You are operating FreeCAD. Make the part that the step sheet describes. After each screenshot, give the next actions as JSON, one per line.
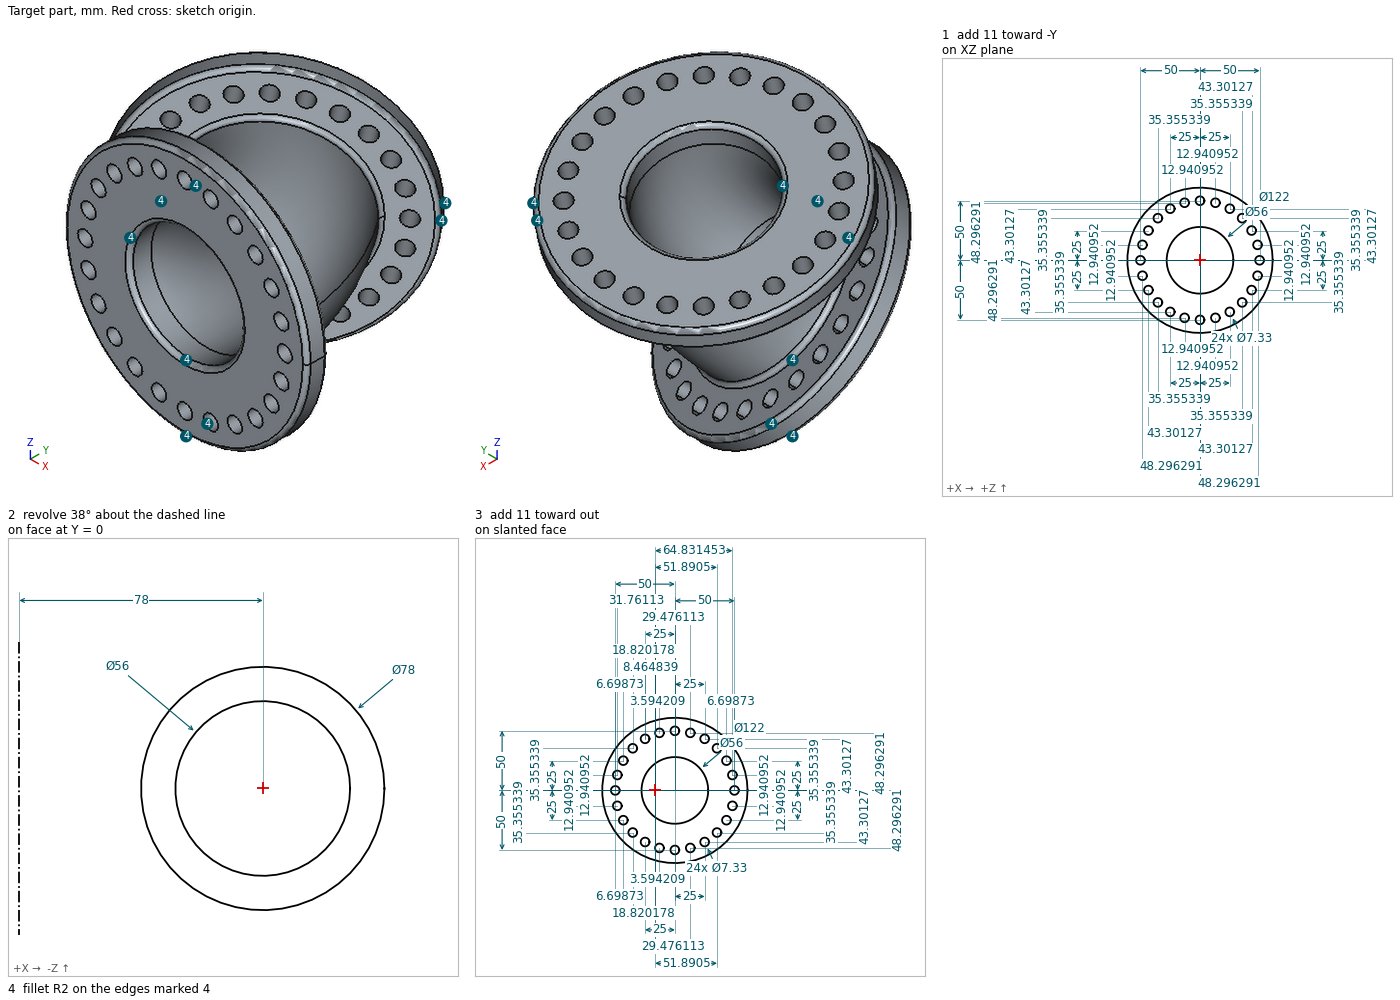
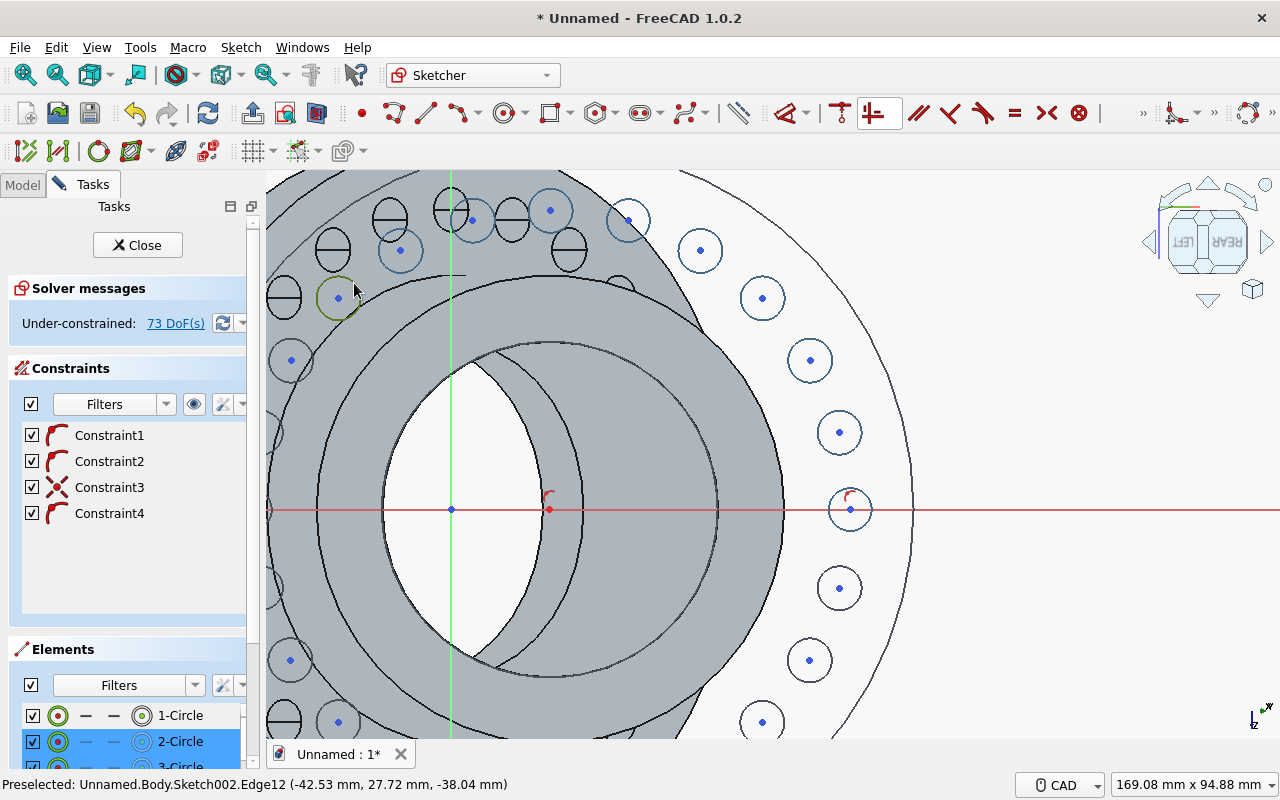
{"action": "left_click", "coordinate": [307, 345]}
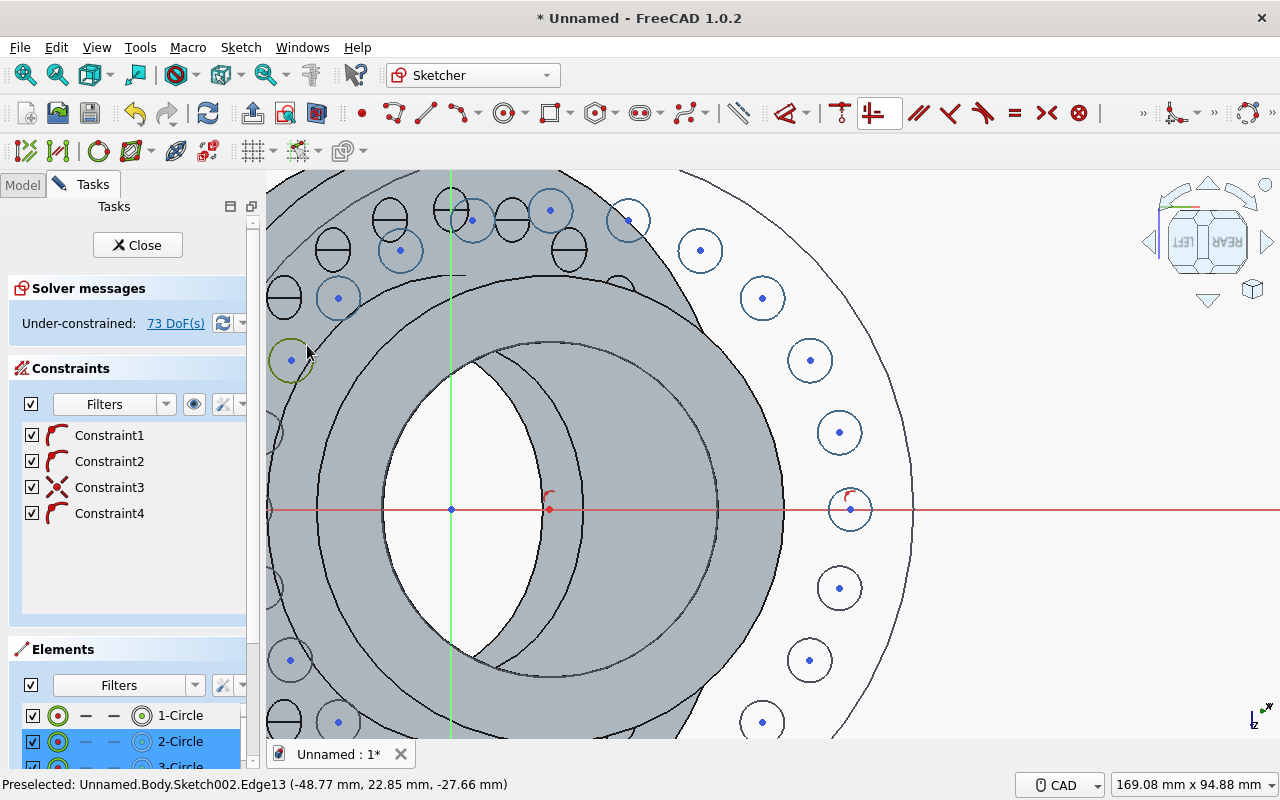
{"action": "scroll", "coordinate": [830, 410], "scroll_direction": "down", "scroll_amount": 4}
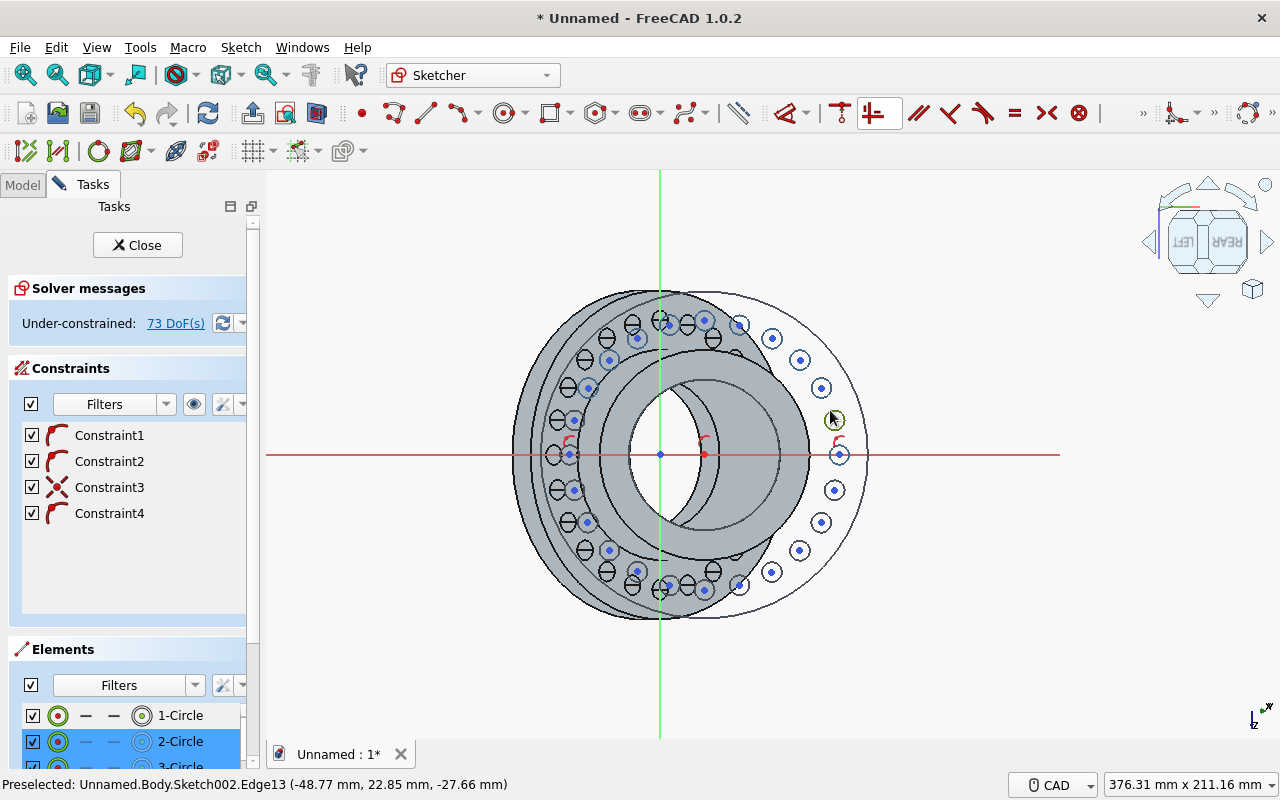
{"action": "scroll", "coordinate": [582, 413], "scroll_direction": "up", "scroll_amount": 2}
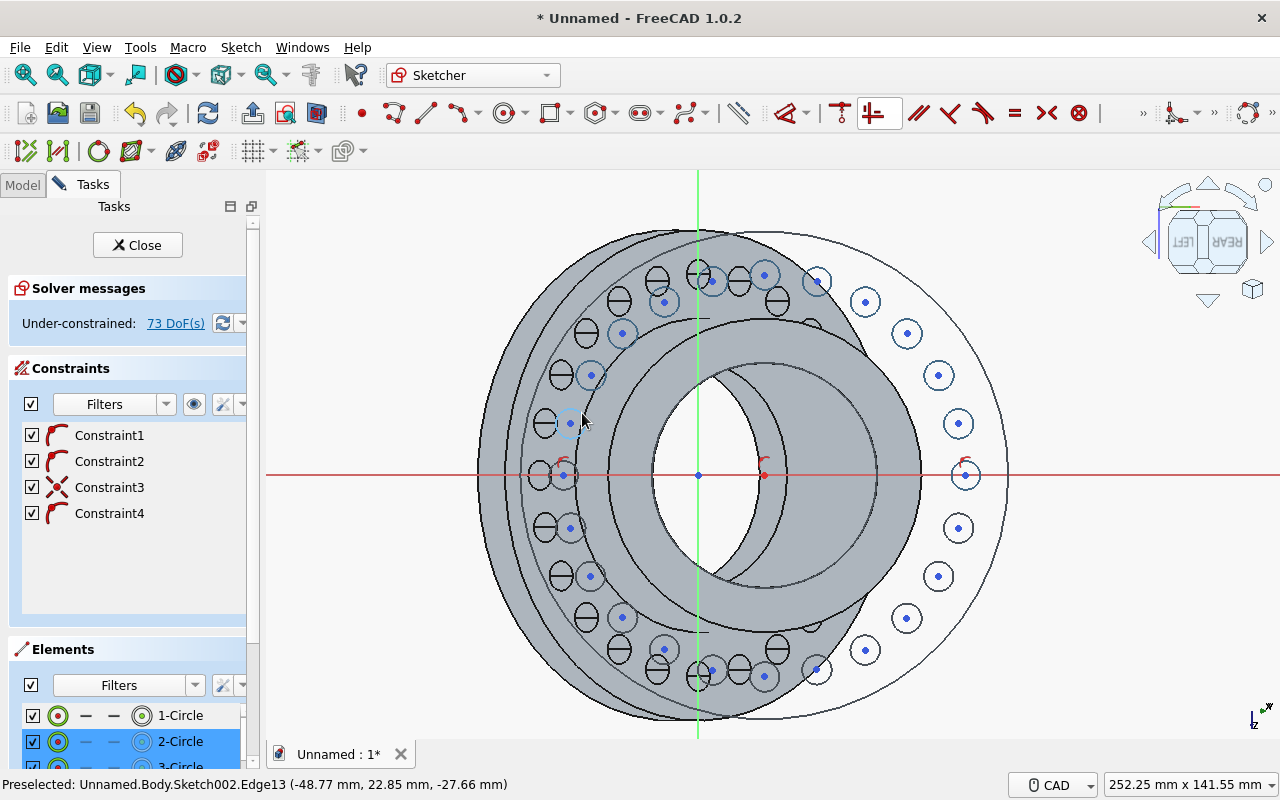
{"action": "left_click", "coordinate": [581, 413]}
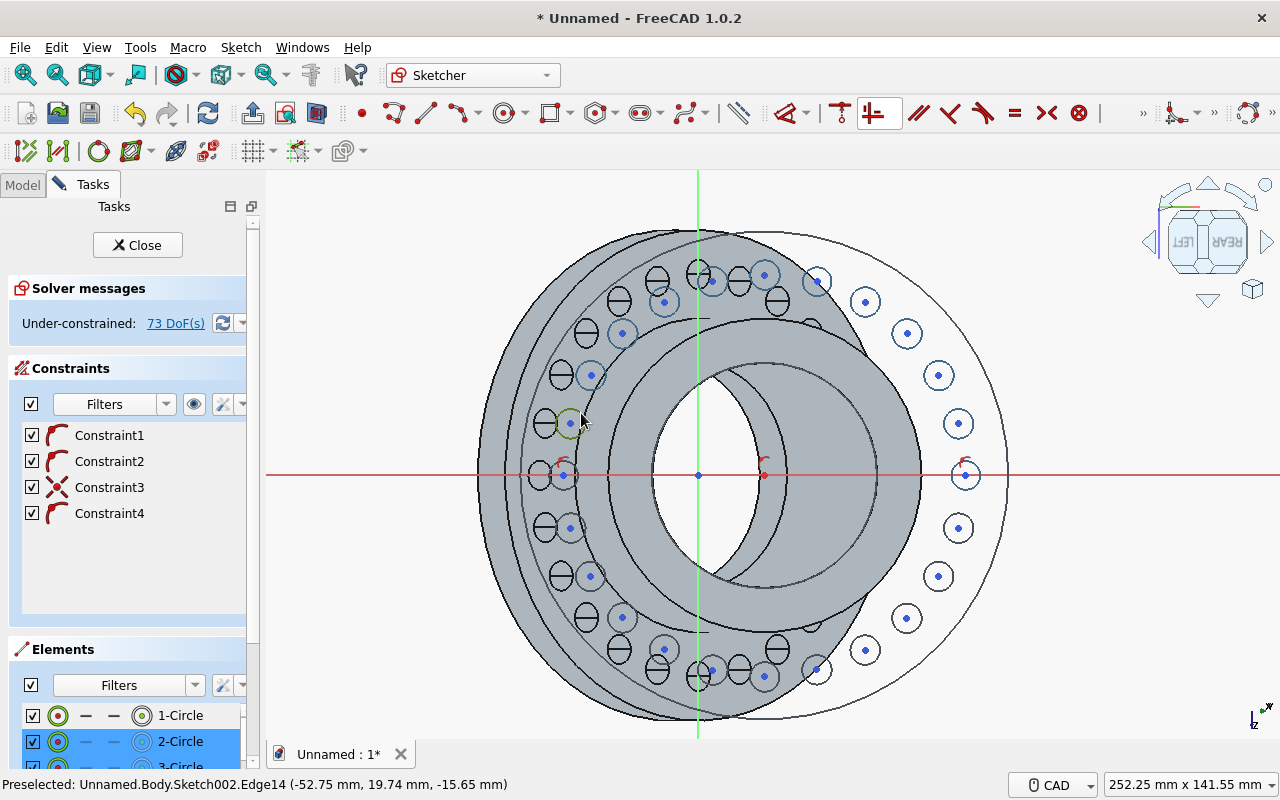
{"action": "left_click", "coordinate": [969, 518]}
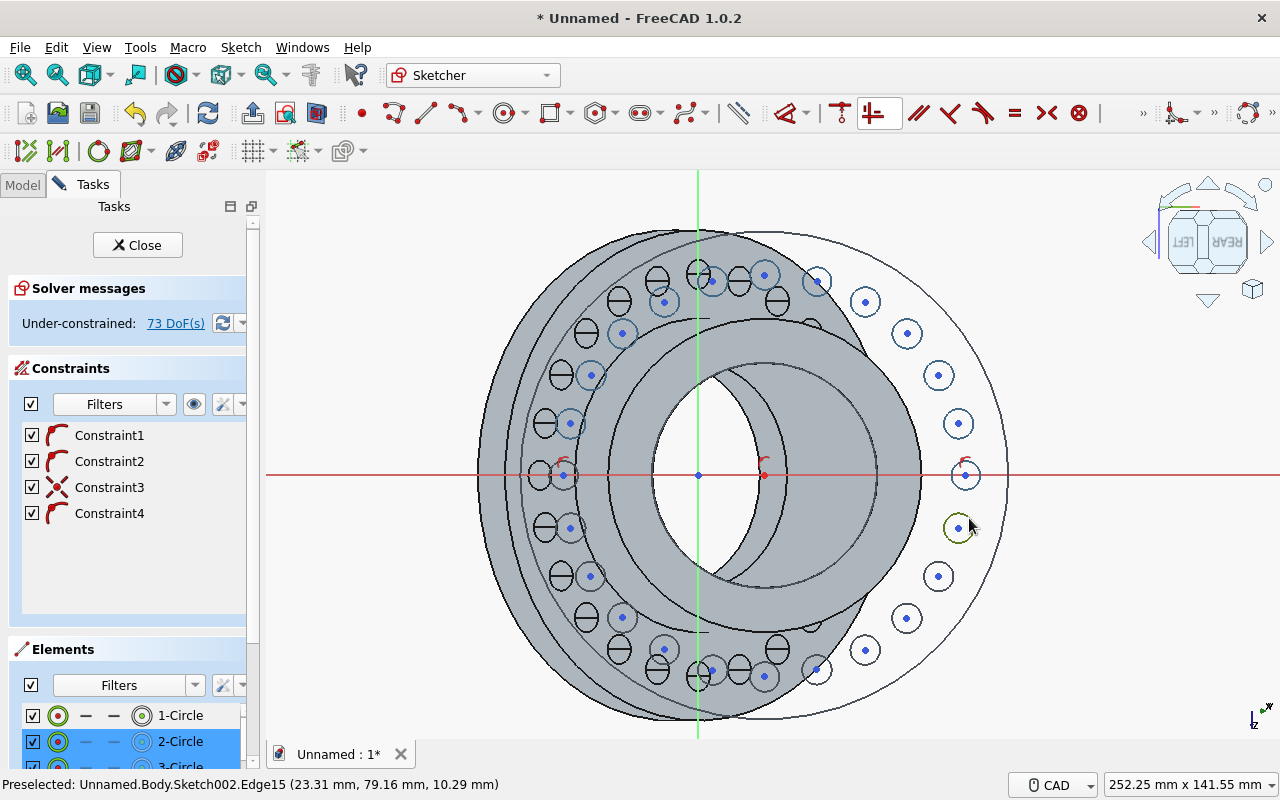
{"action": "left_click", "coordinate": [949, 566]}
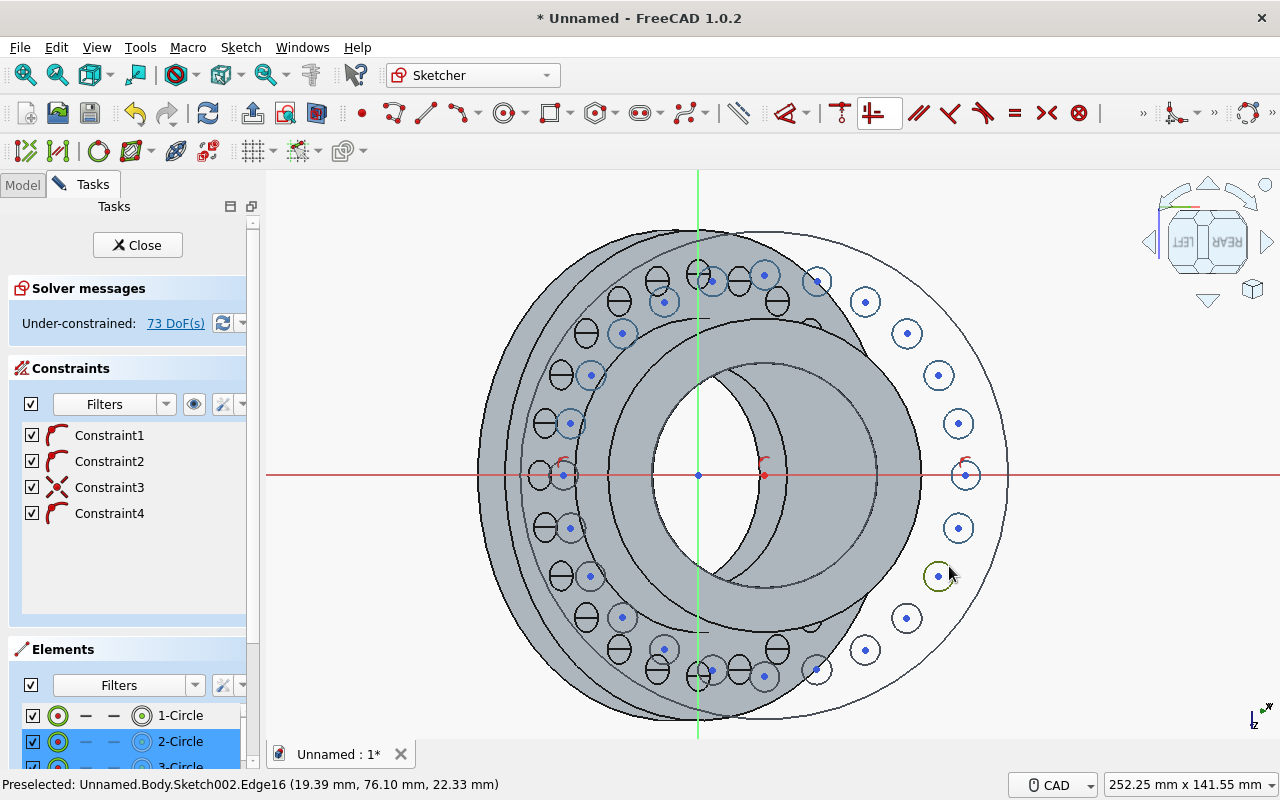
{"action": "left_click", "coordinate": [917, 608]}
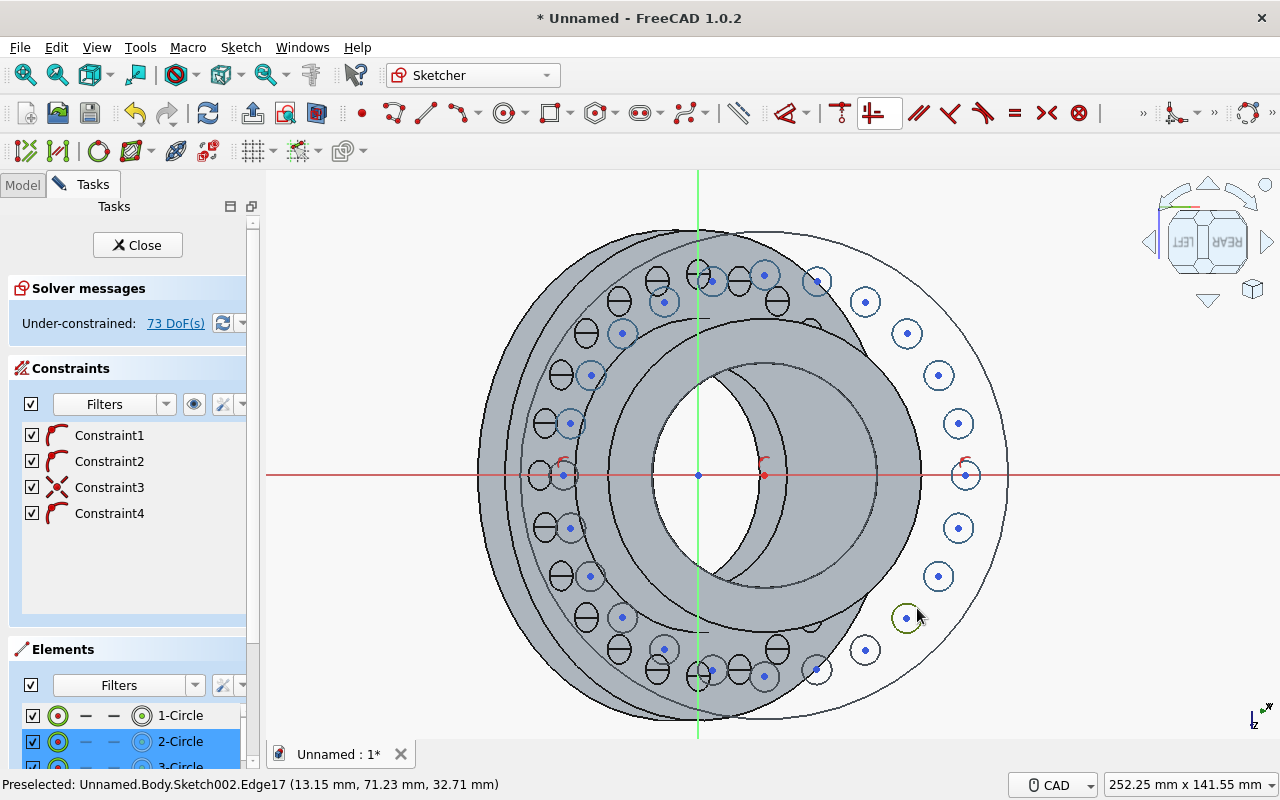
{"action": "left_click", "coordinate": [876, 640]}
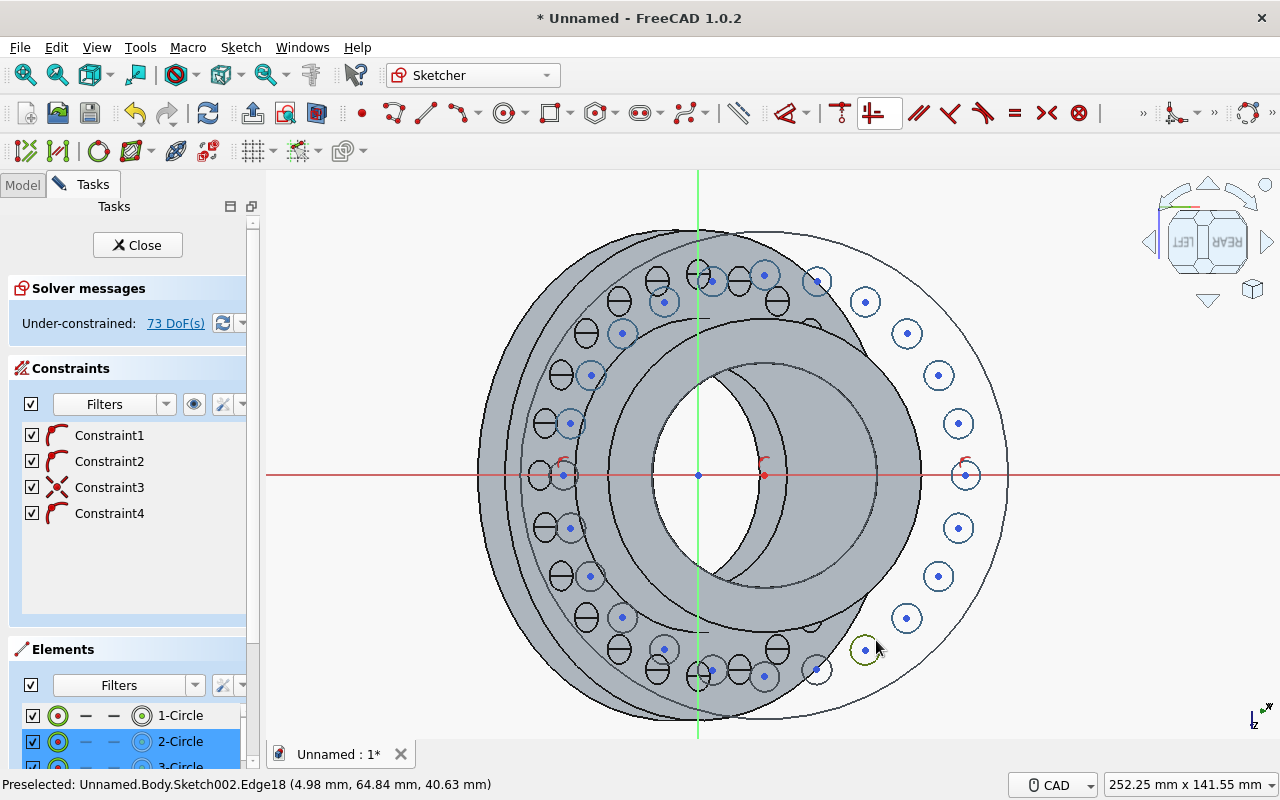
{"action": "left_click", "coordinate": [827, 659]}